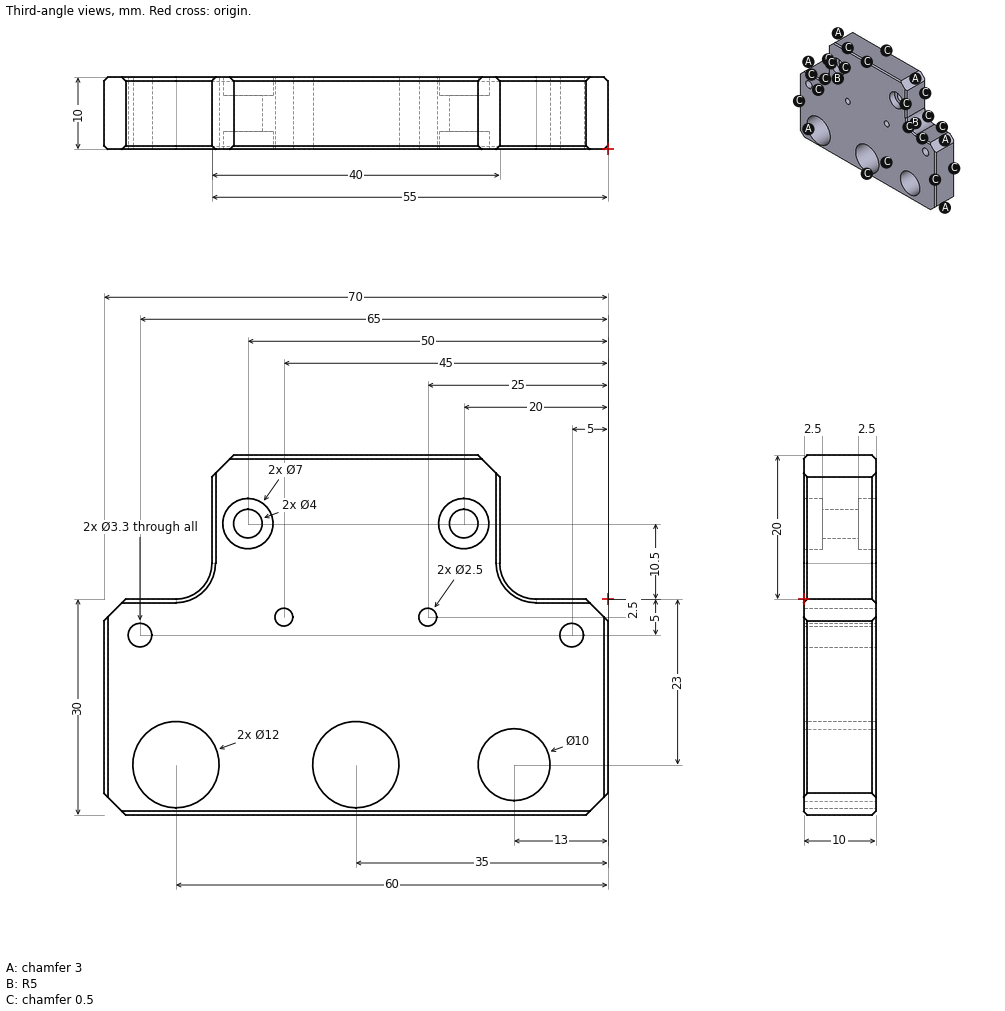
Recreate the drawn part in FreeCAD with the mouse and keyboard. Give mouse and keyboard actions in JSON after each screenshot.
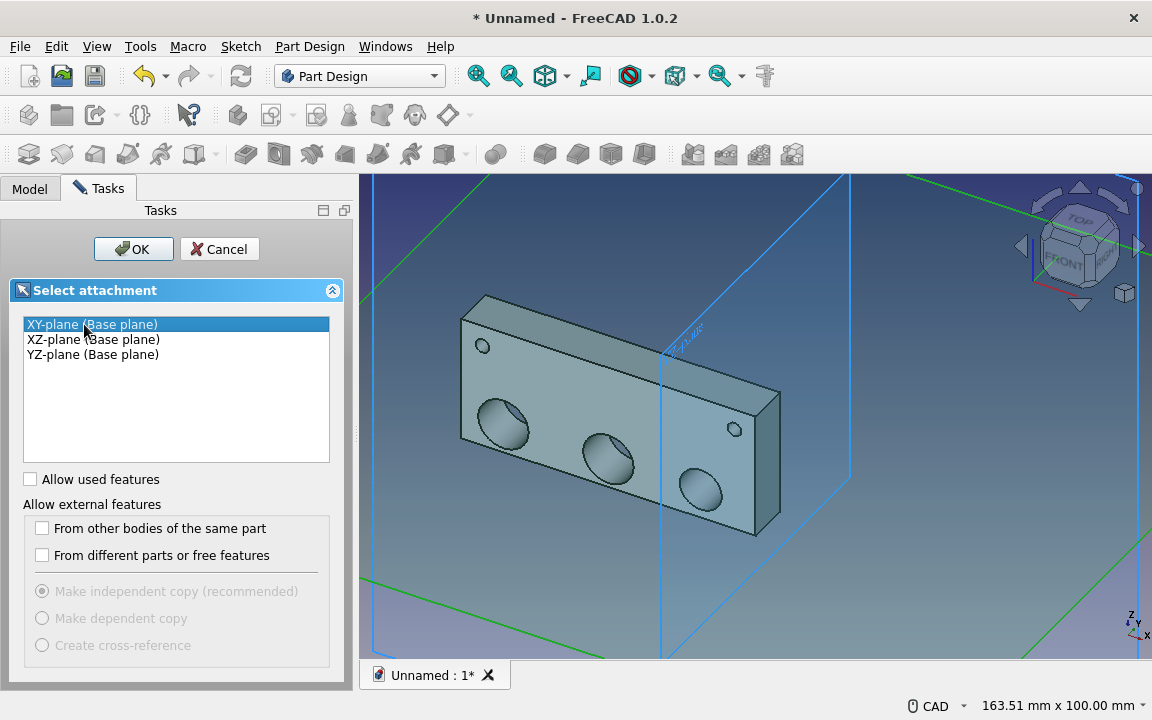
{"action": "left_click", "coordinate": [134, 249]}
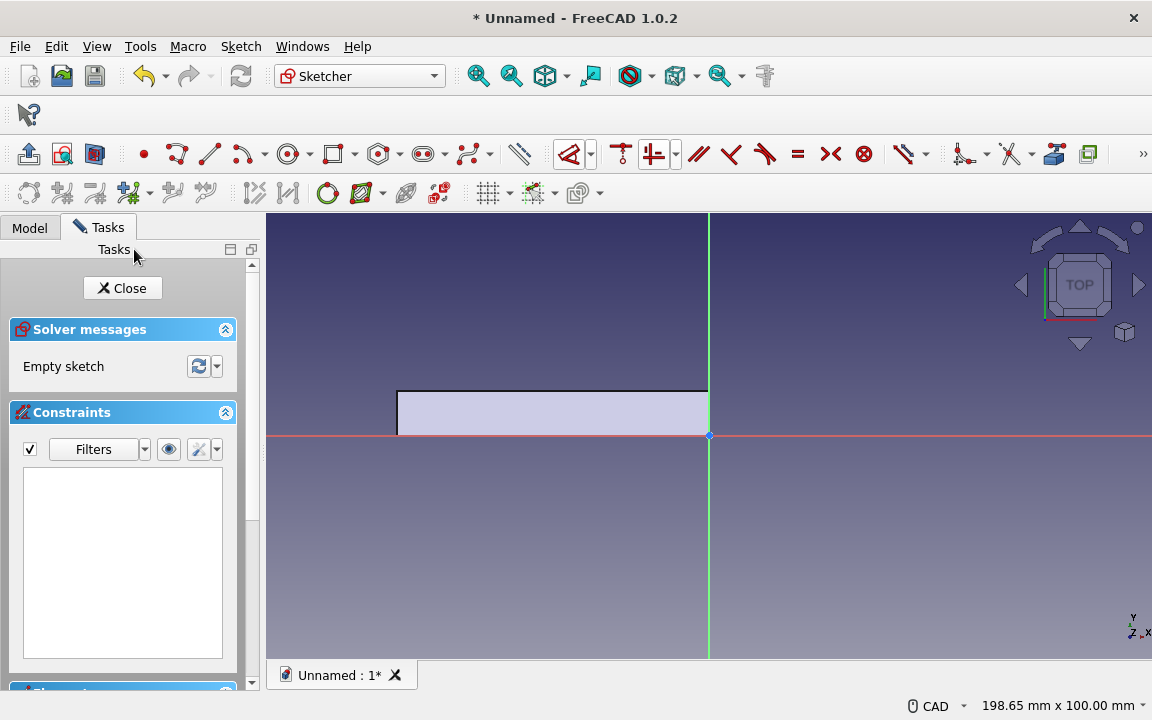
{"action": "scroll", "coordinate": [520, 387], "scroll_direction": "up", "scroll_amount": 3}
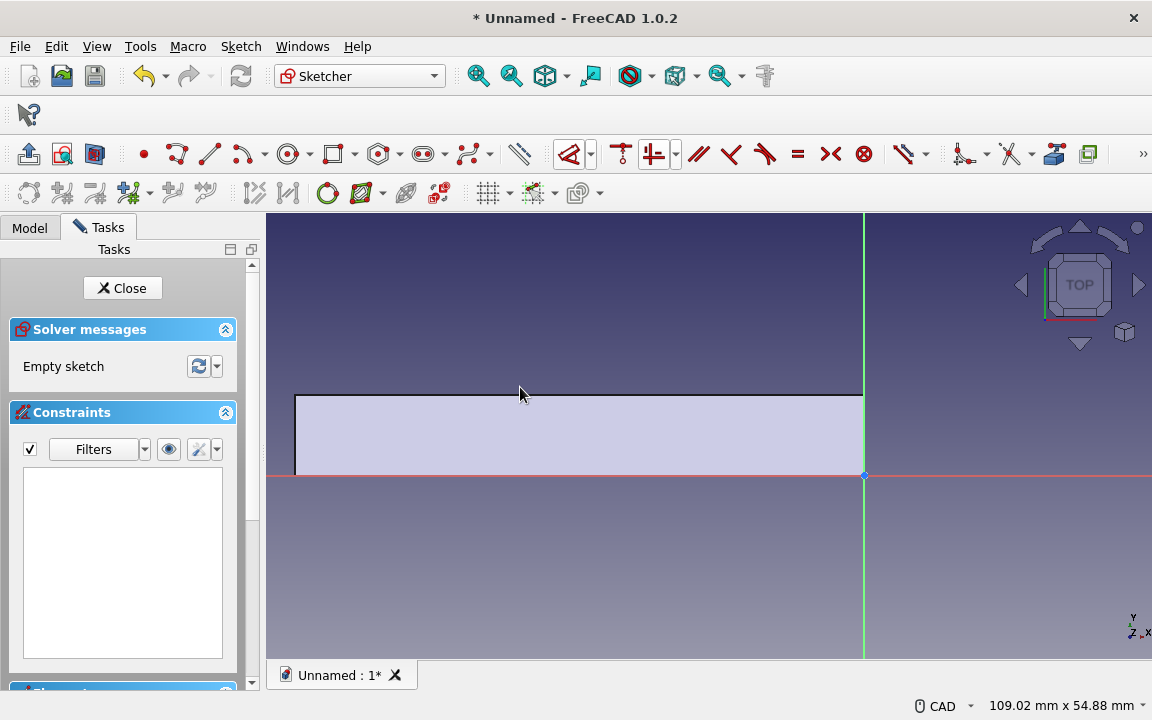
{"action": "left_click", "coordinate": [332, 154]}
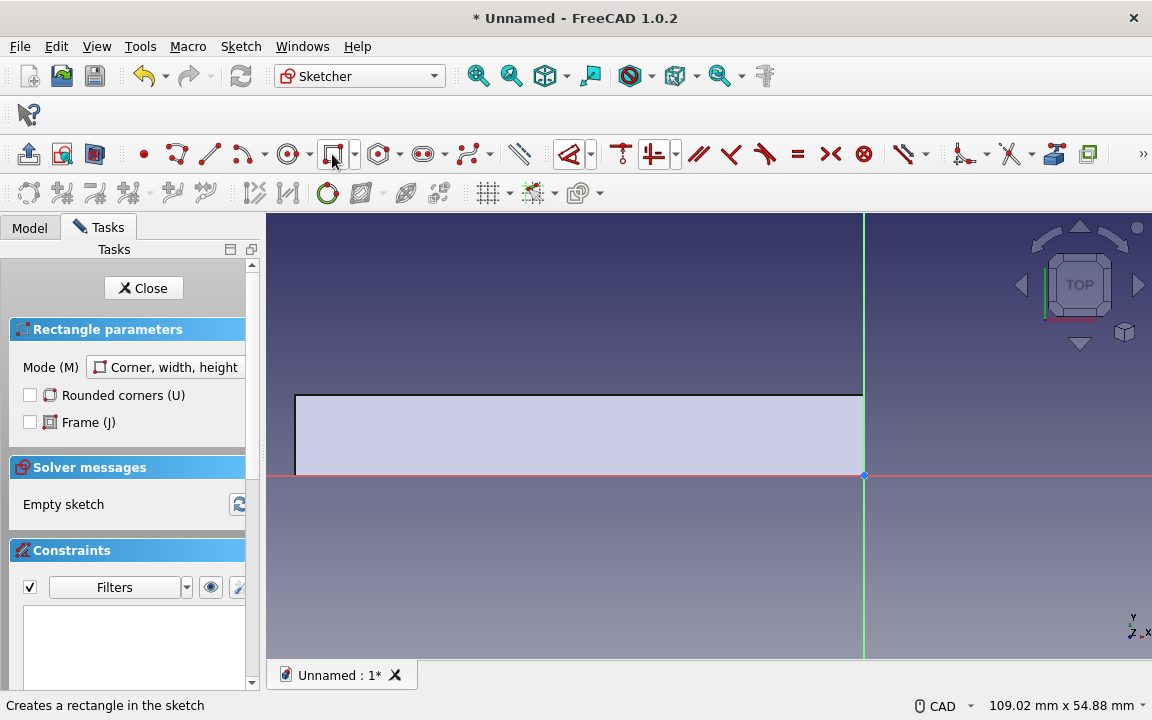
{"action": "left_click", "coordinate": [417, 395]}
{"action": "left_click", "coordinate": [742, 476]}
{"action": "key", "text": "Escape"}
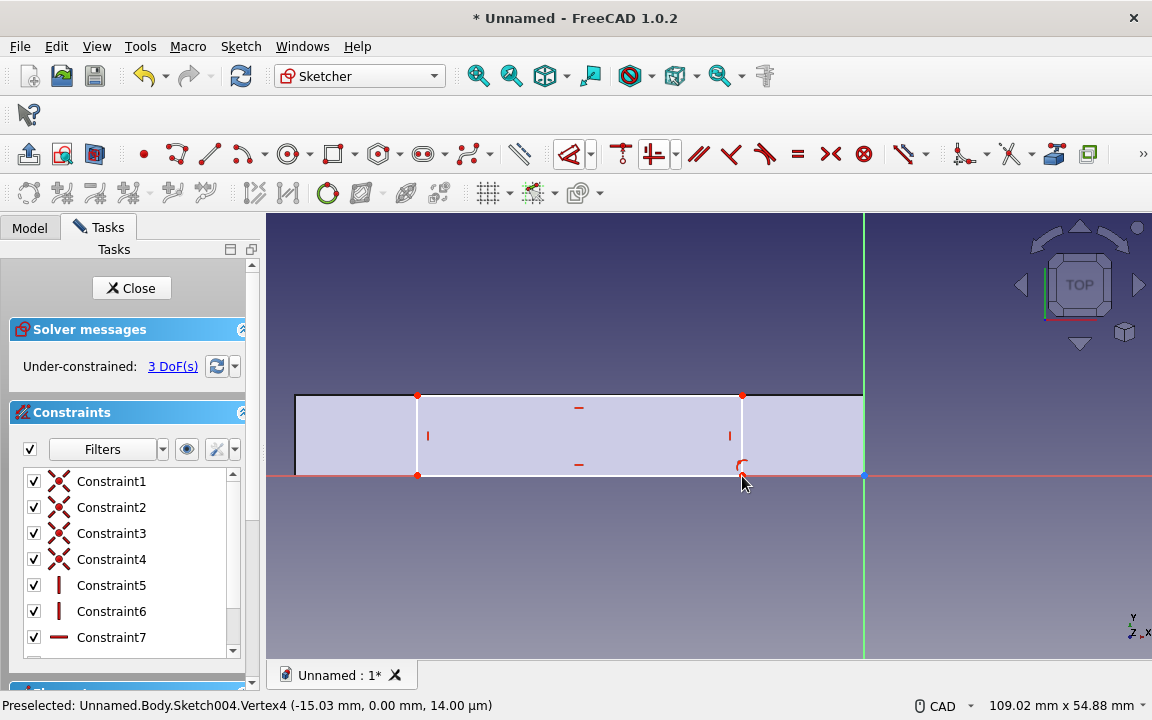
{"action": "left_click", "coordinate": [417, 420]}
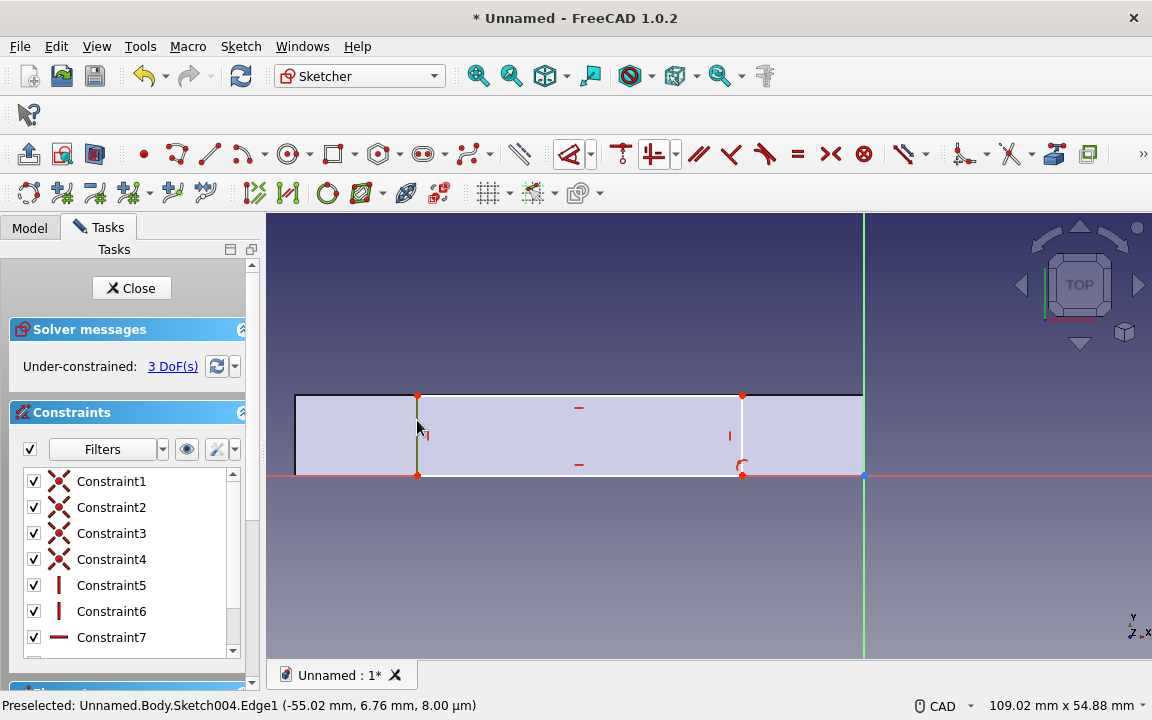
{"action": "left_click", "coordinate": [590, 154]}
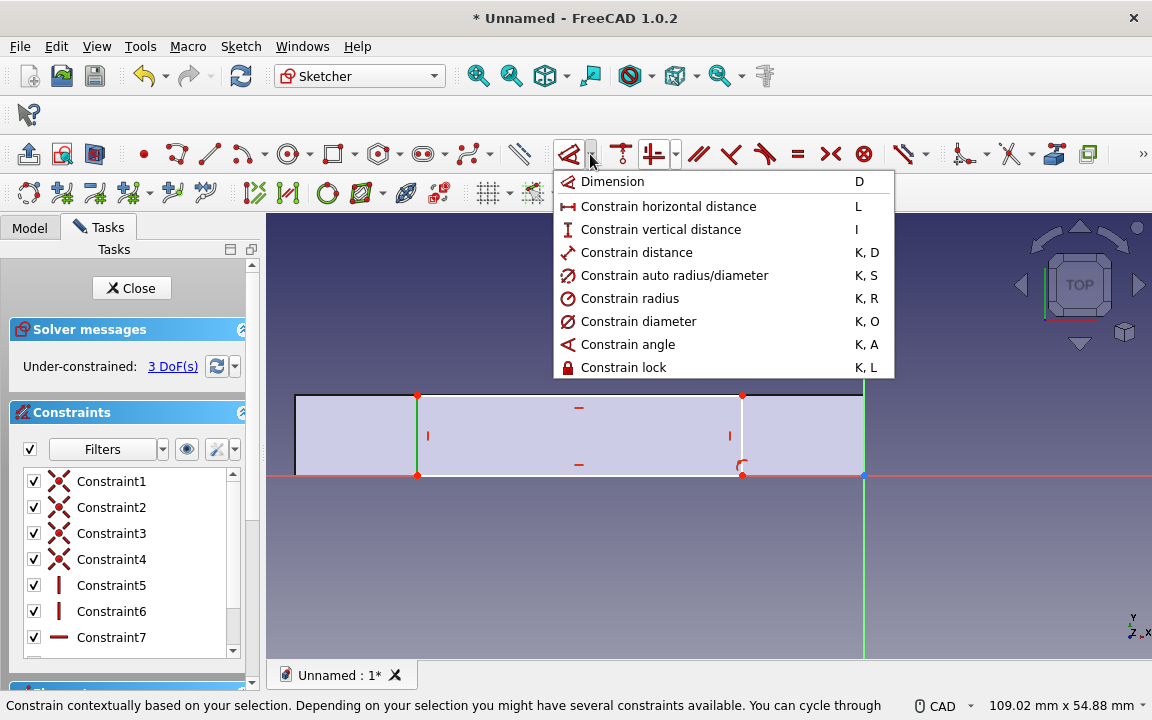
{"action": "left_click", "coordinate": [724, 230]}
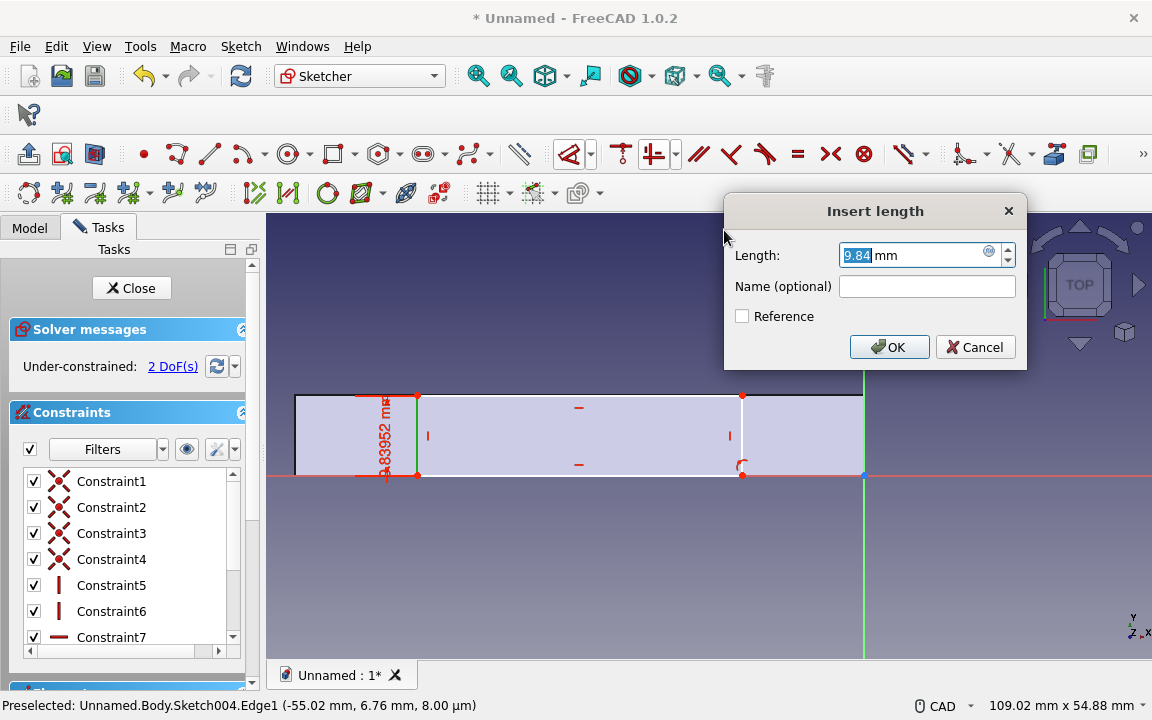
{"action": "type", "text": "10"}
{"action": "key", "text": "Return"}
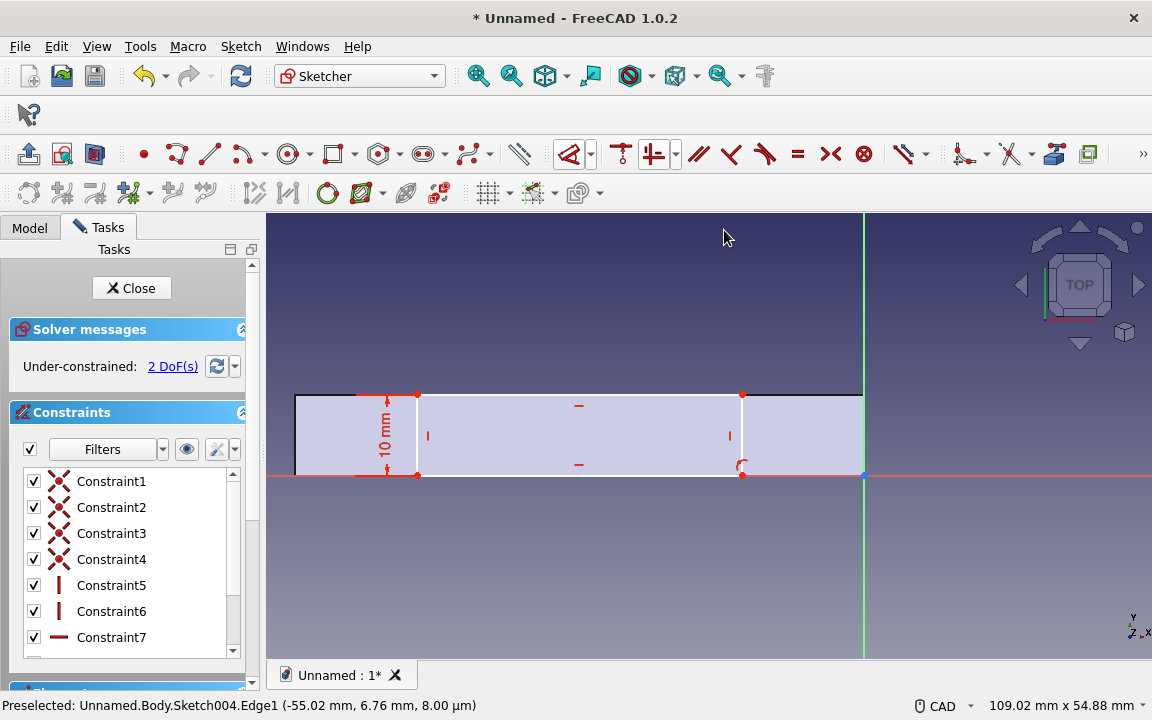
{"action": "left_click", "coordinate": [514, 476]}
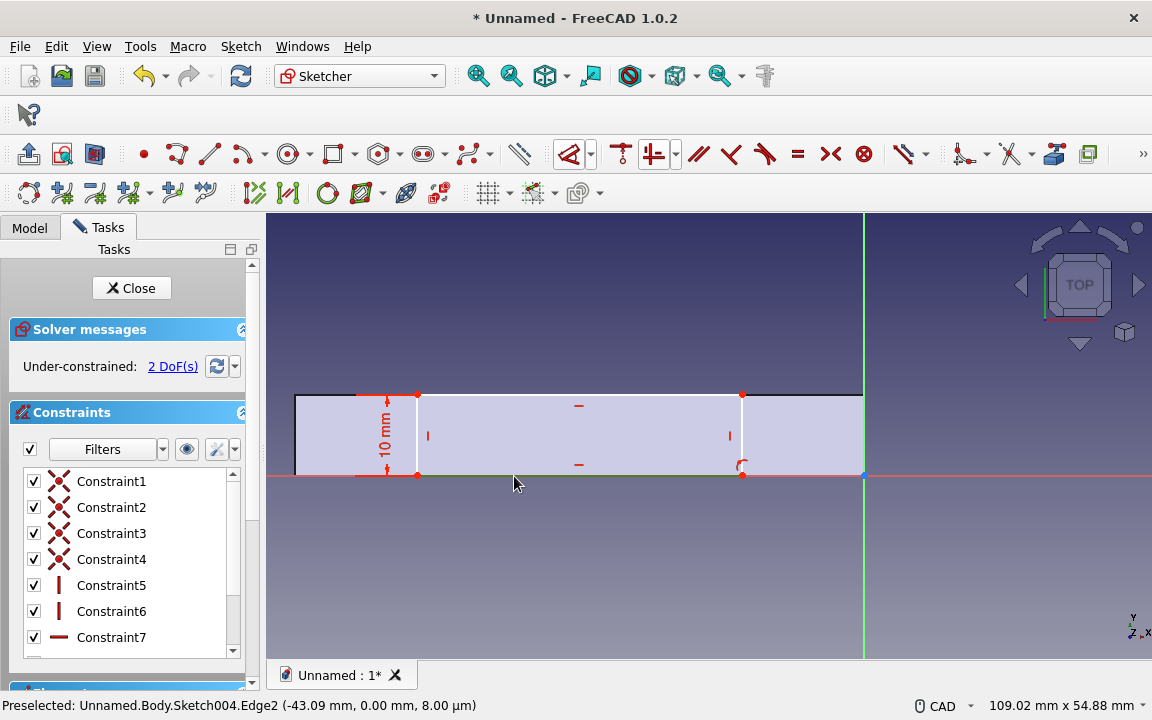
{"action": "left_click", "coordinate": [590, 154]}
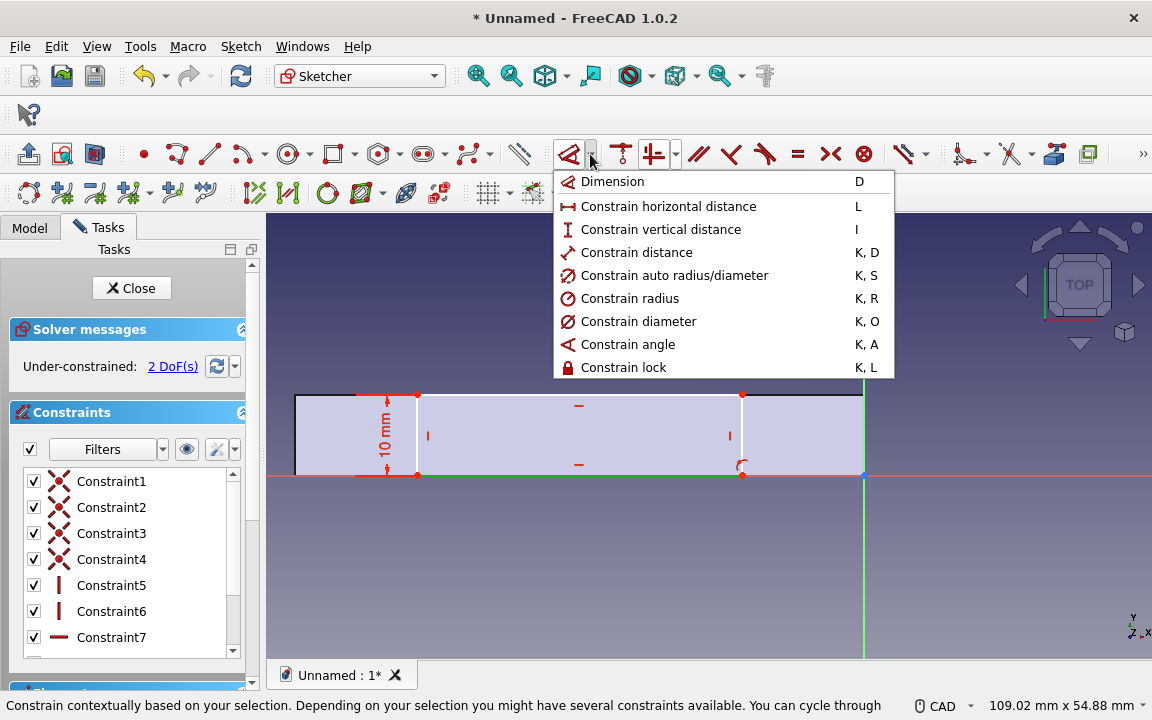
{"action": "left_click", "coordinate": [724, 206]}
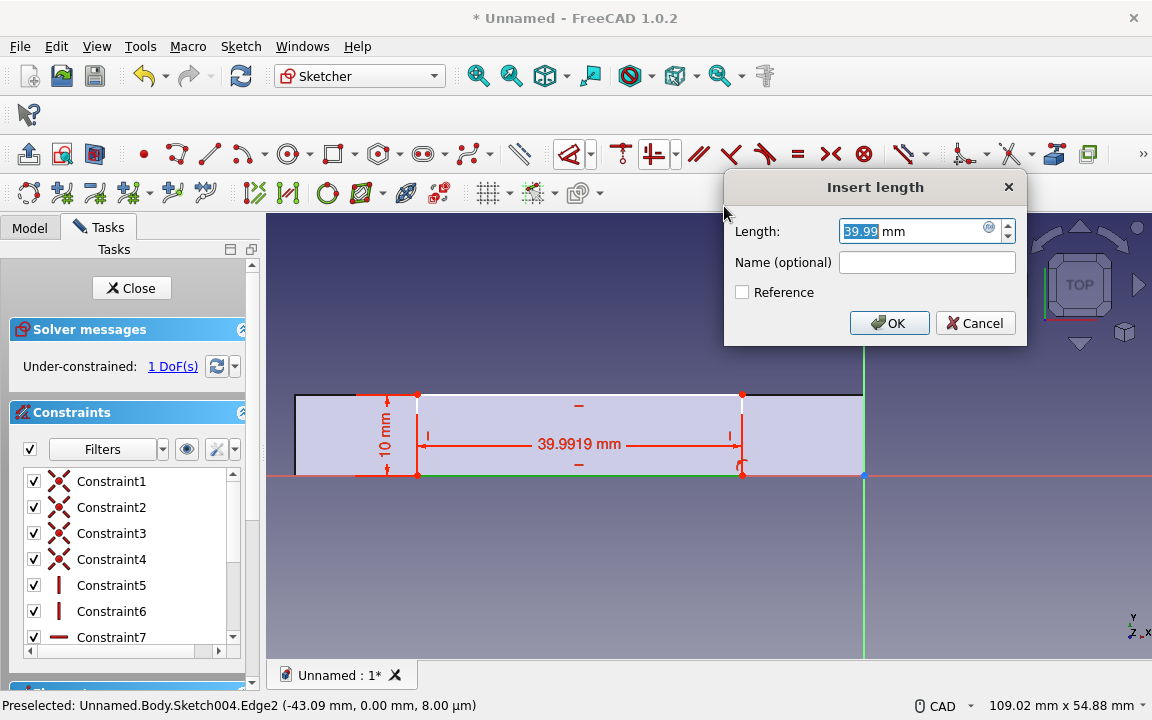
{"action": "type", "text": "40"}
{"action": "key", "text": "Return"}